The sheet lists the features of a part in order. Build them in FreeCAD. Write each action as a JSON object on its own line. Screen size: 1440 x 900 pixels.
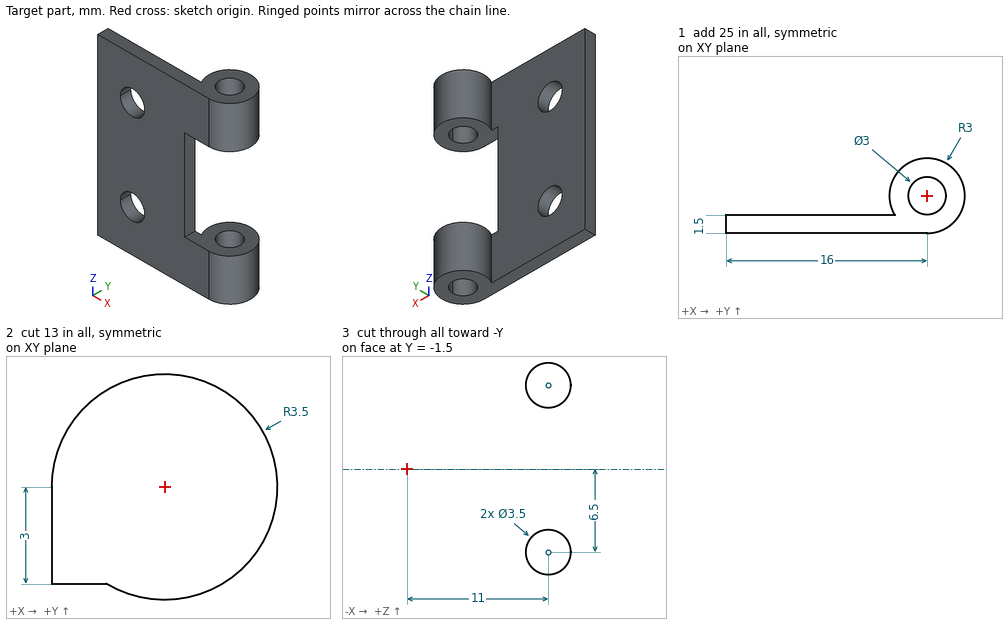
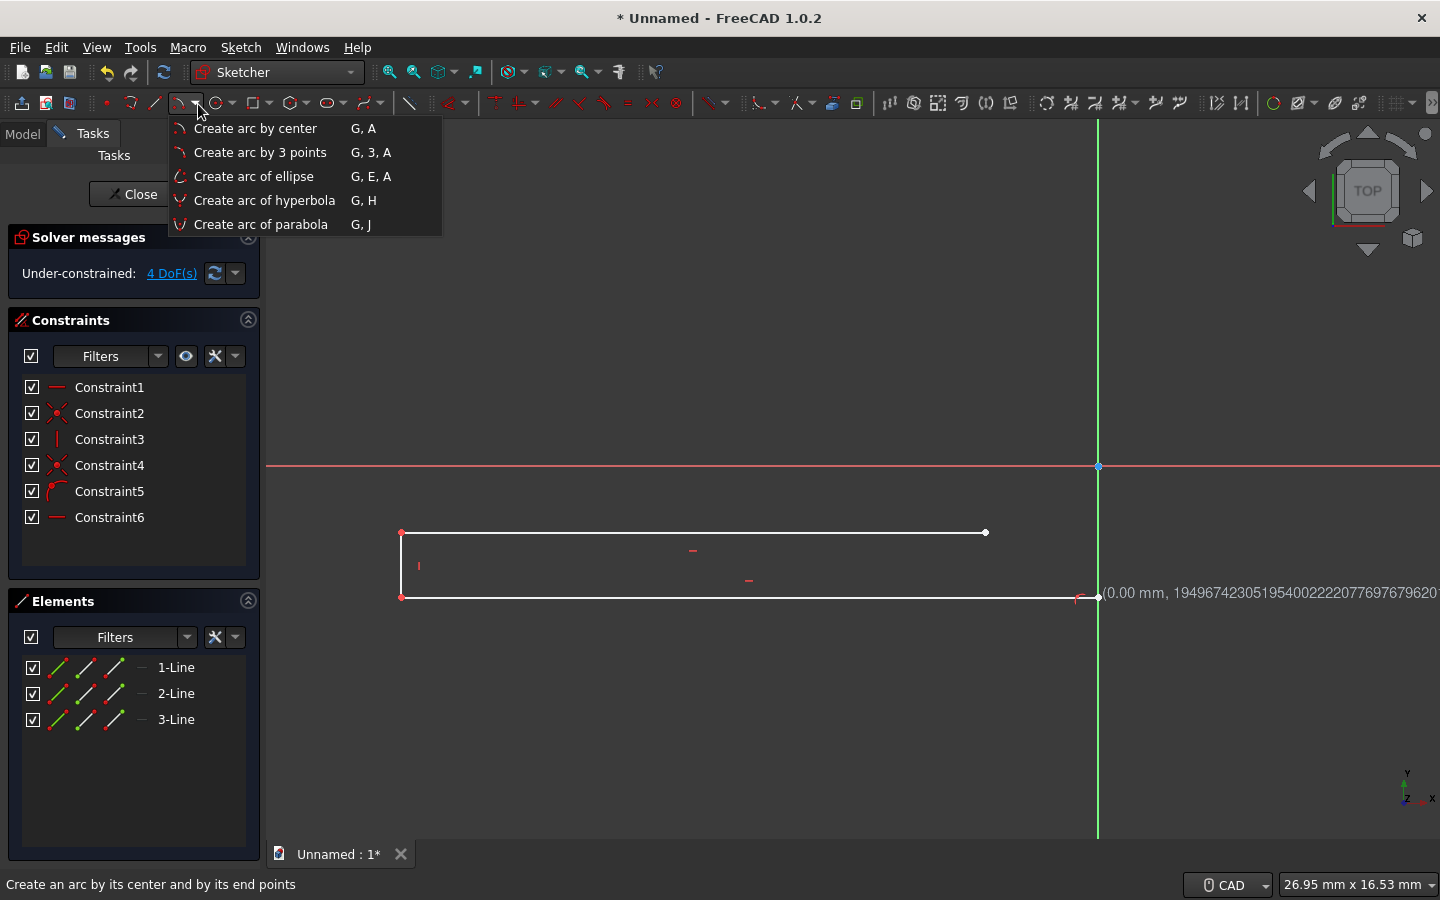
{"action": "left_click", "coordinate": [306, 152]}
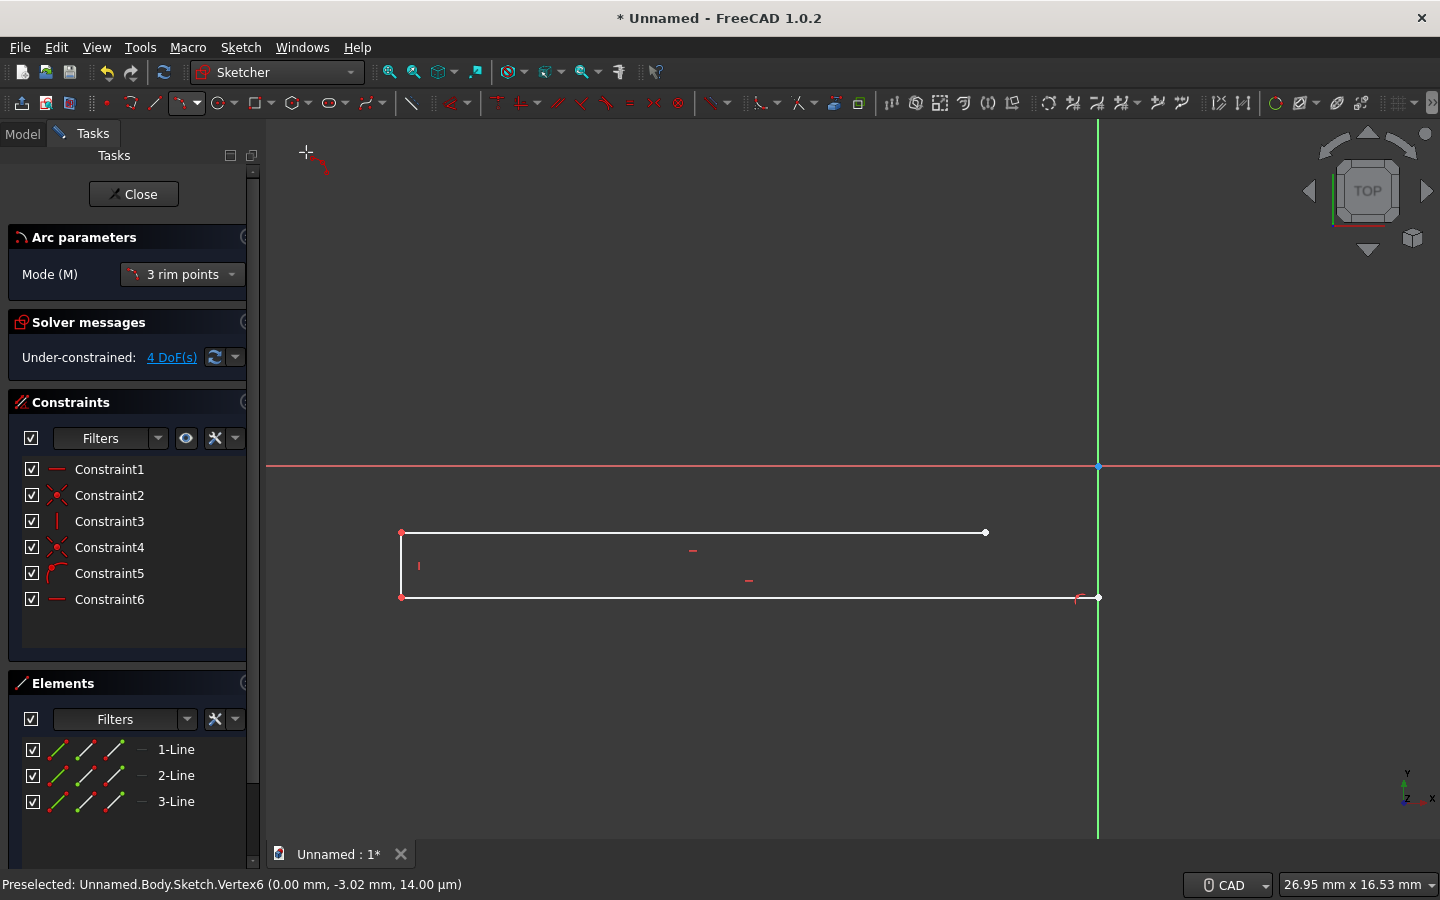
{"action": "left_click", "coordinate": [1098, 598]}
{"action": "left_click", "coordinate": [985, 533]}
{"action": "left_click", "coordinate": [1163, 353]}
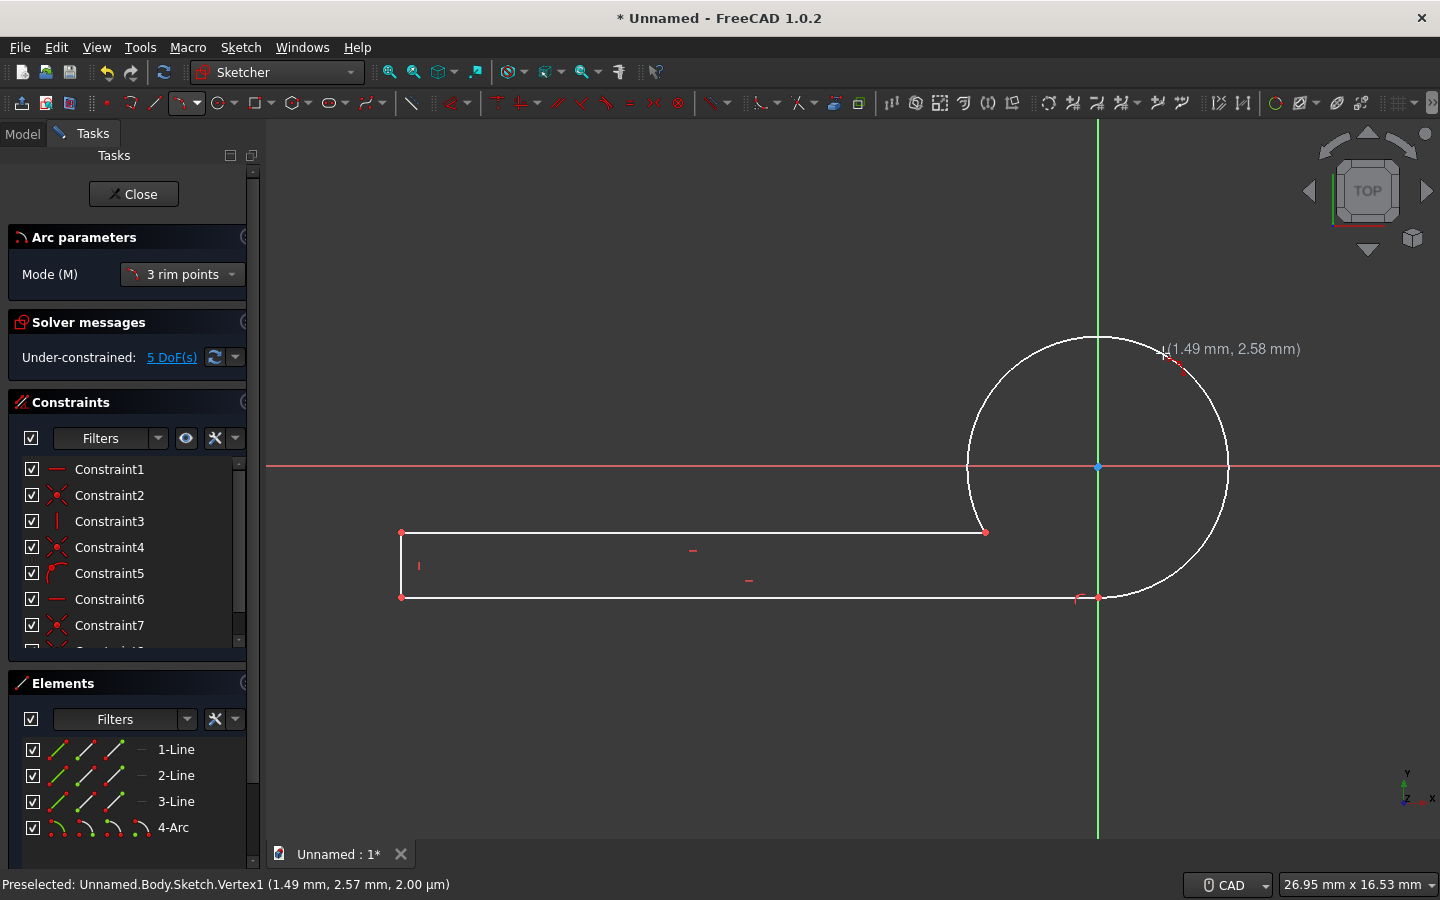
{"action": "left_click", "coordinate": [218, 104]}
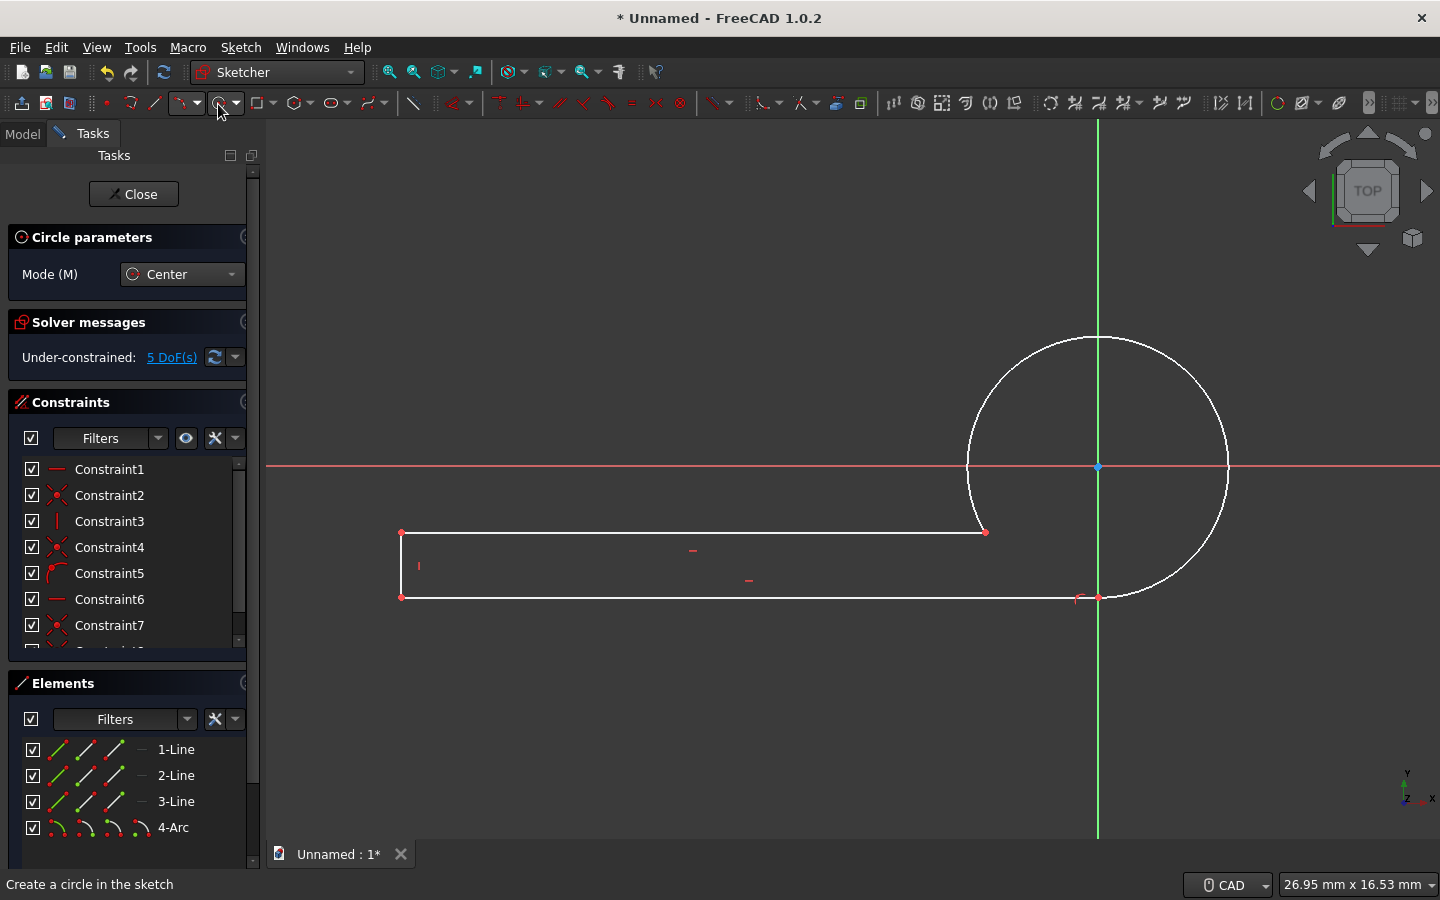
{"action": "left_click", "coordinate": [1098, 466]}
{"action": "left_click", "coordinate": [1144, 420]}
{"action": "key", "text": "Escape"}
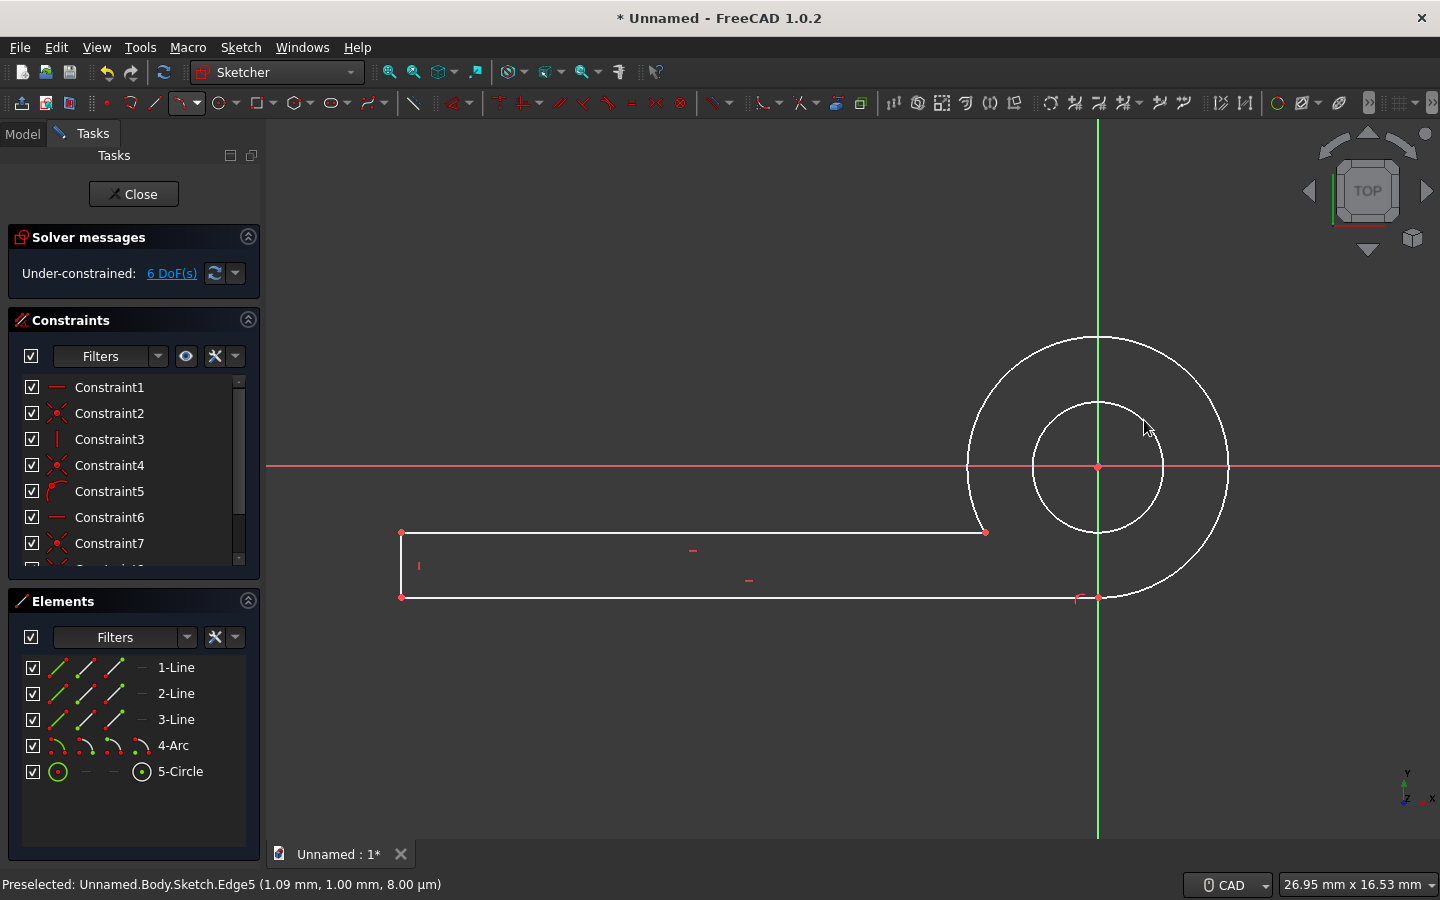
{"action": "left_click", "coordinate": [610, 598]}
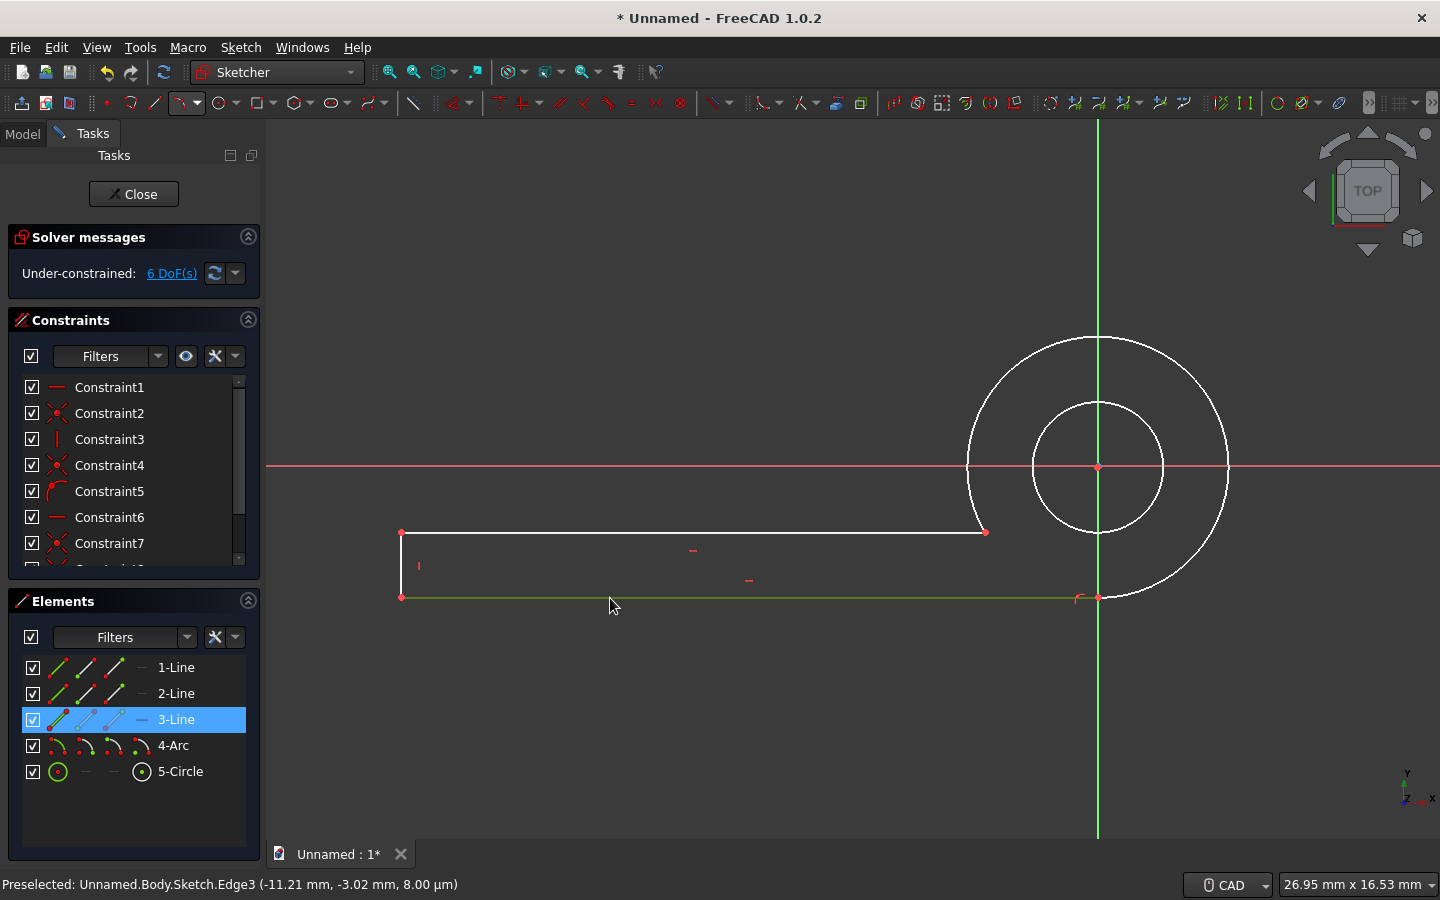
{"action": "left_click", "coordinate": [1229, 467]}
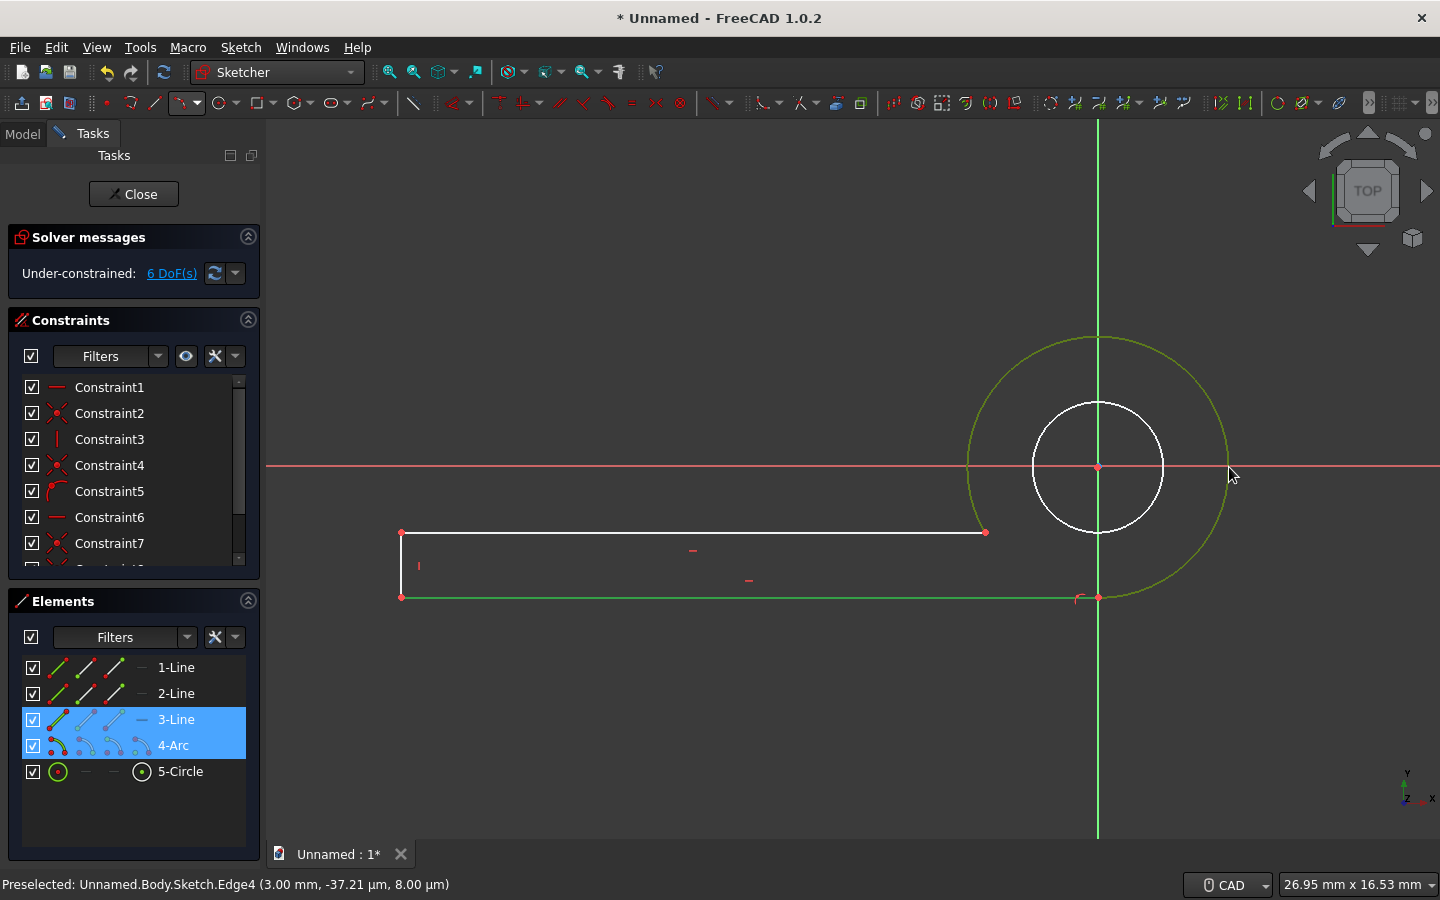
{"action": "left_click", "coordinate": [608, 104]}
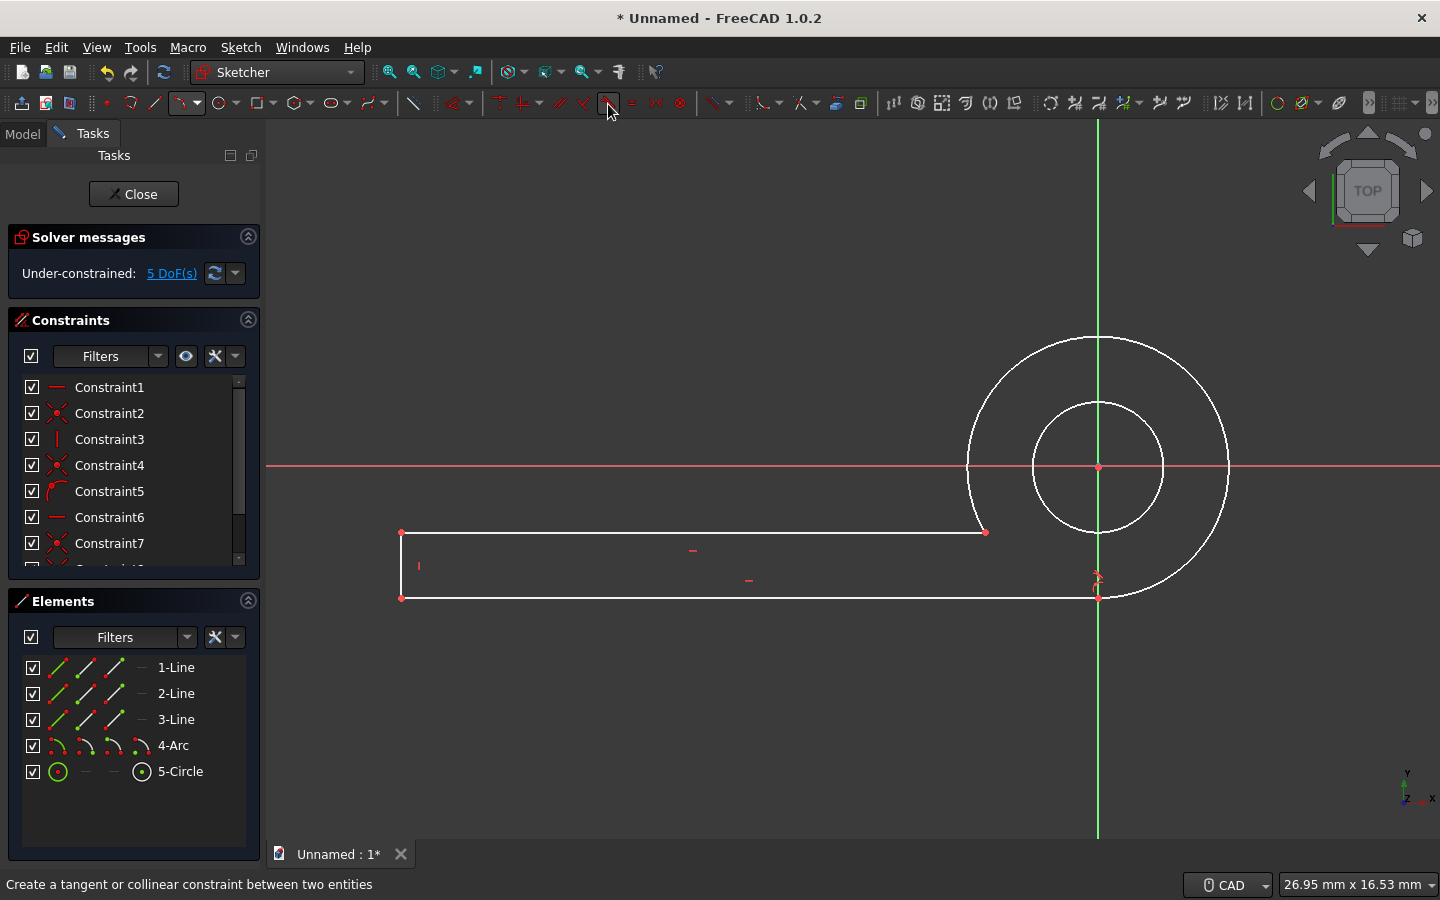
{"action": "left_click", "coordinate": [1098, 467]}